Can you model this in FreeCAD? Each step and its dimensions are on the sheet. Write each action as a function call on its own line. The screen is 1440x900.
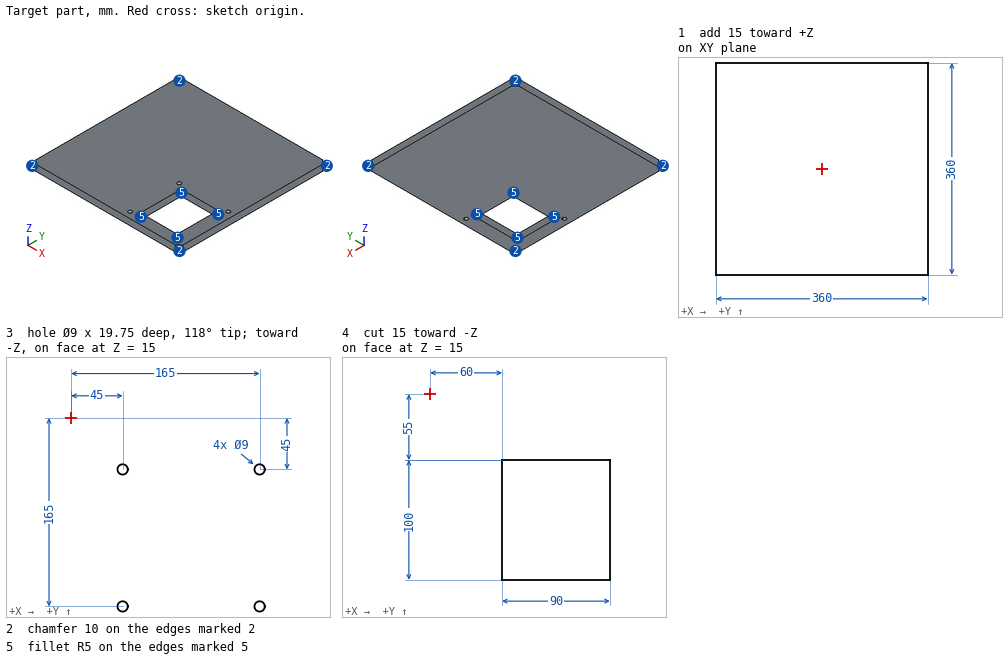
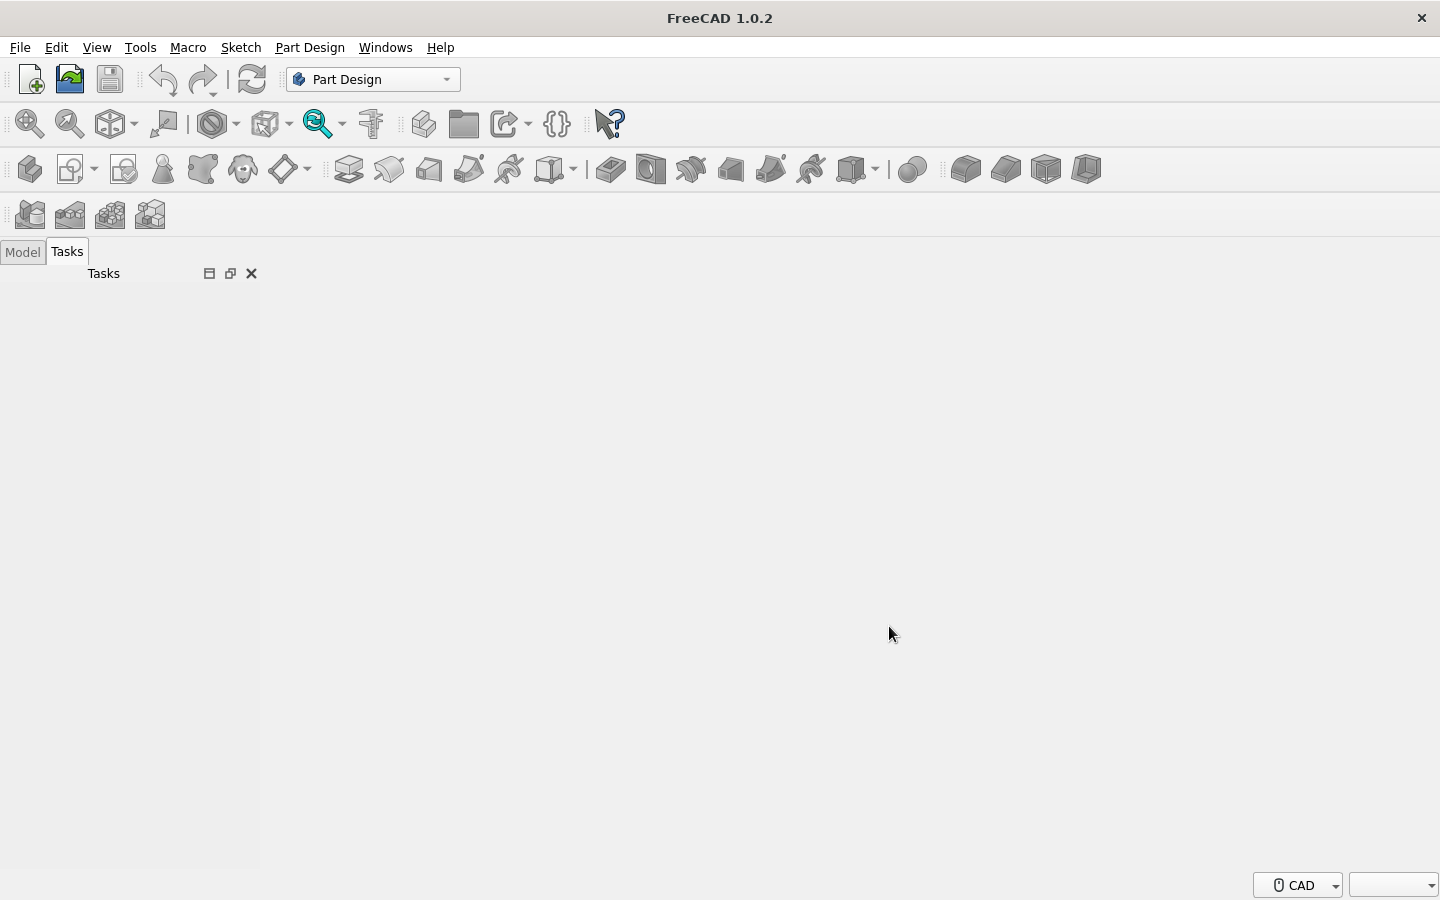
key(ctrl+n)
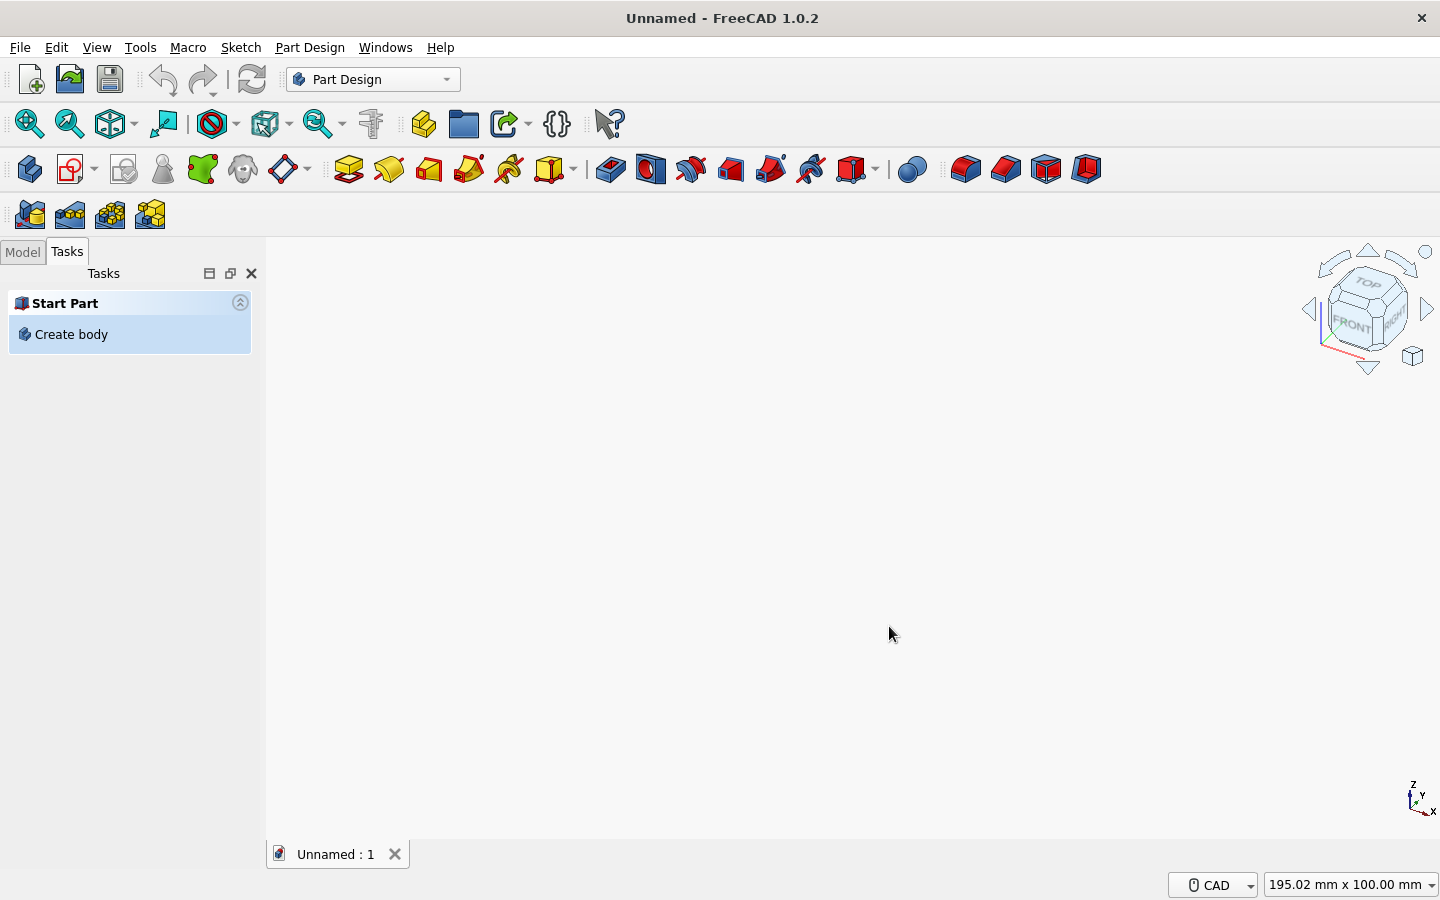
click(70, 170)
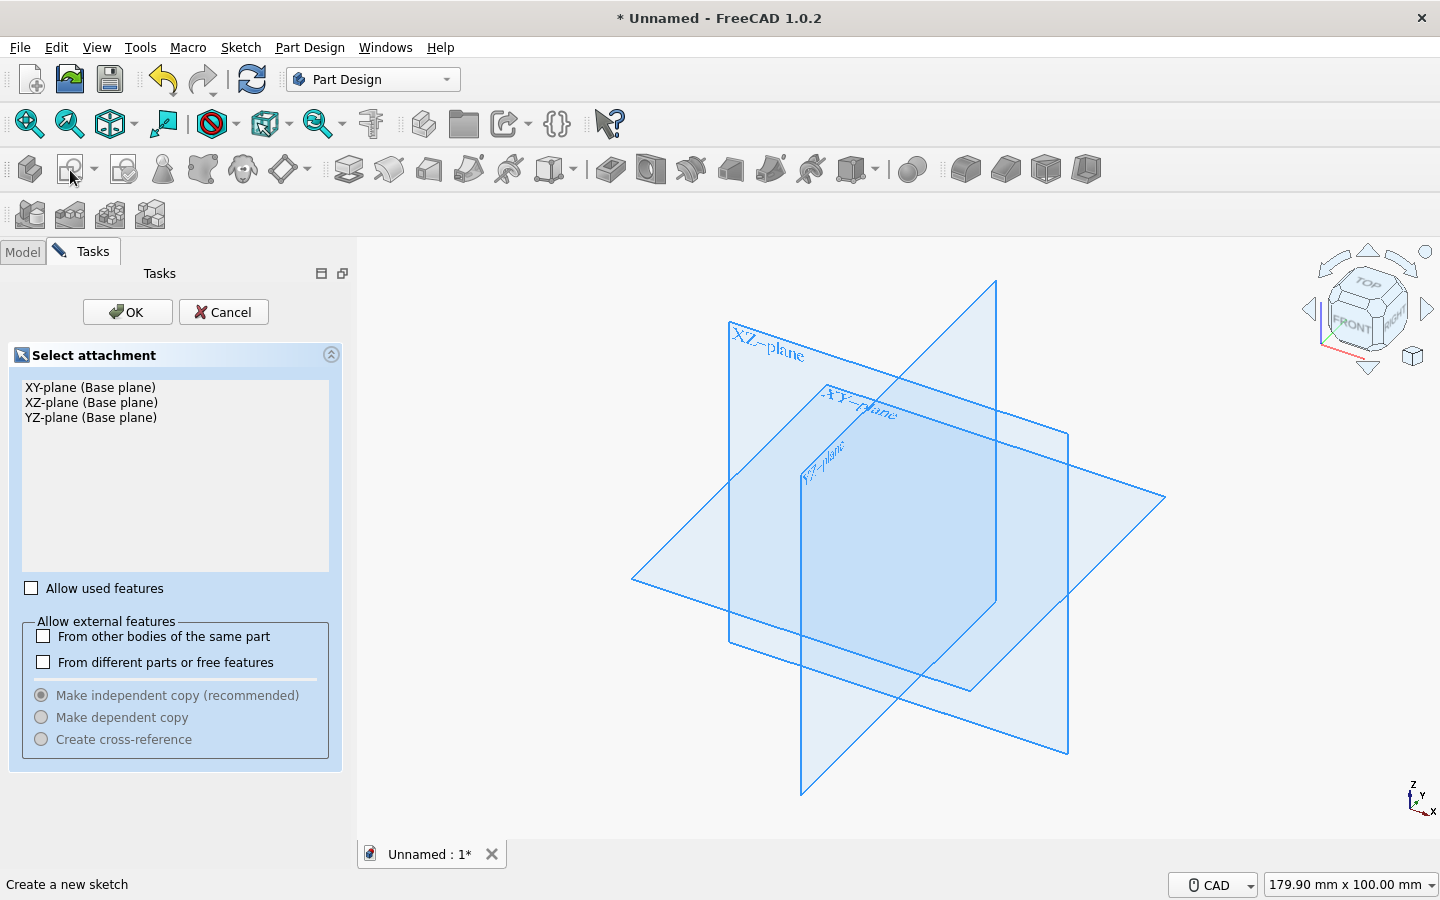
click(82, 388)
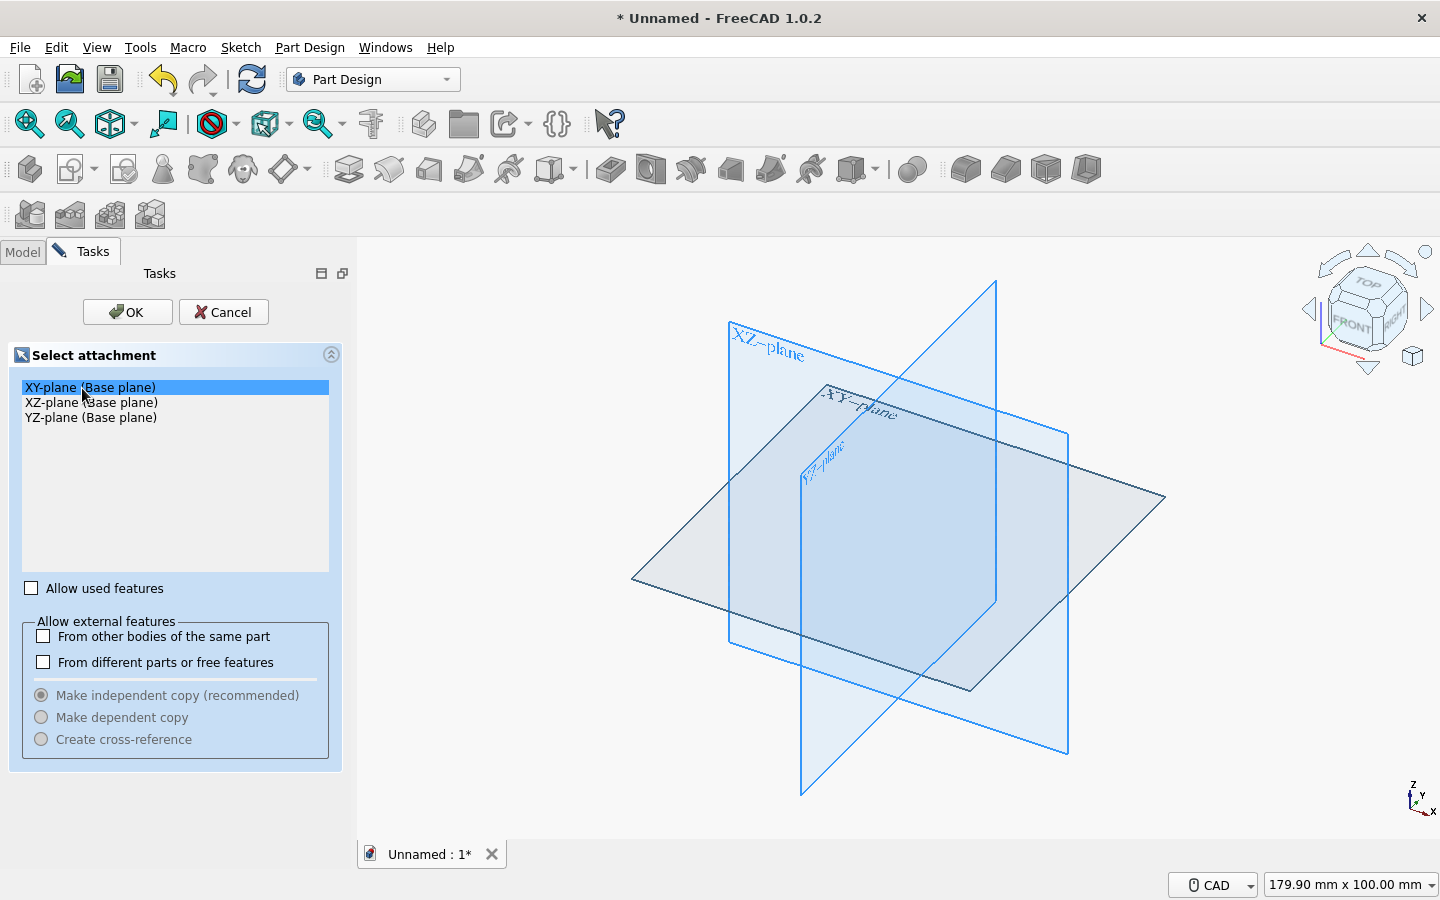
click(128, 312)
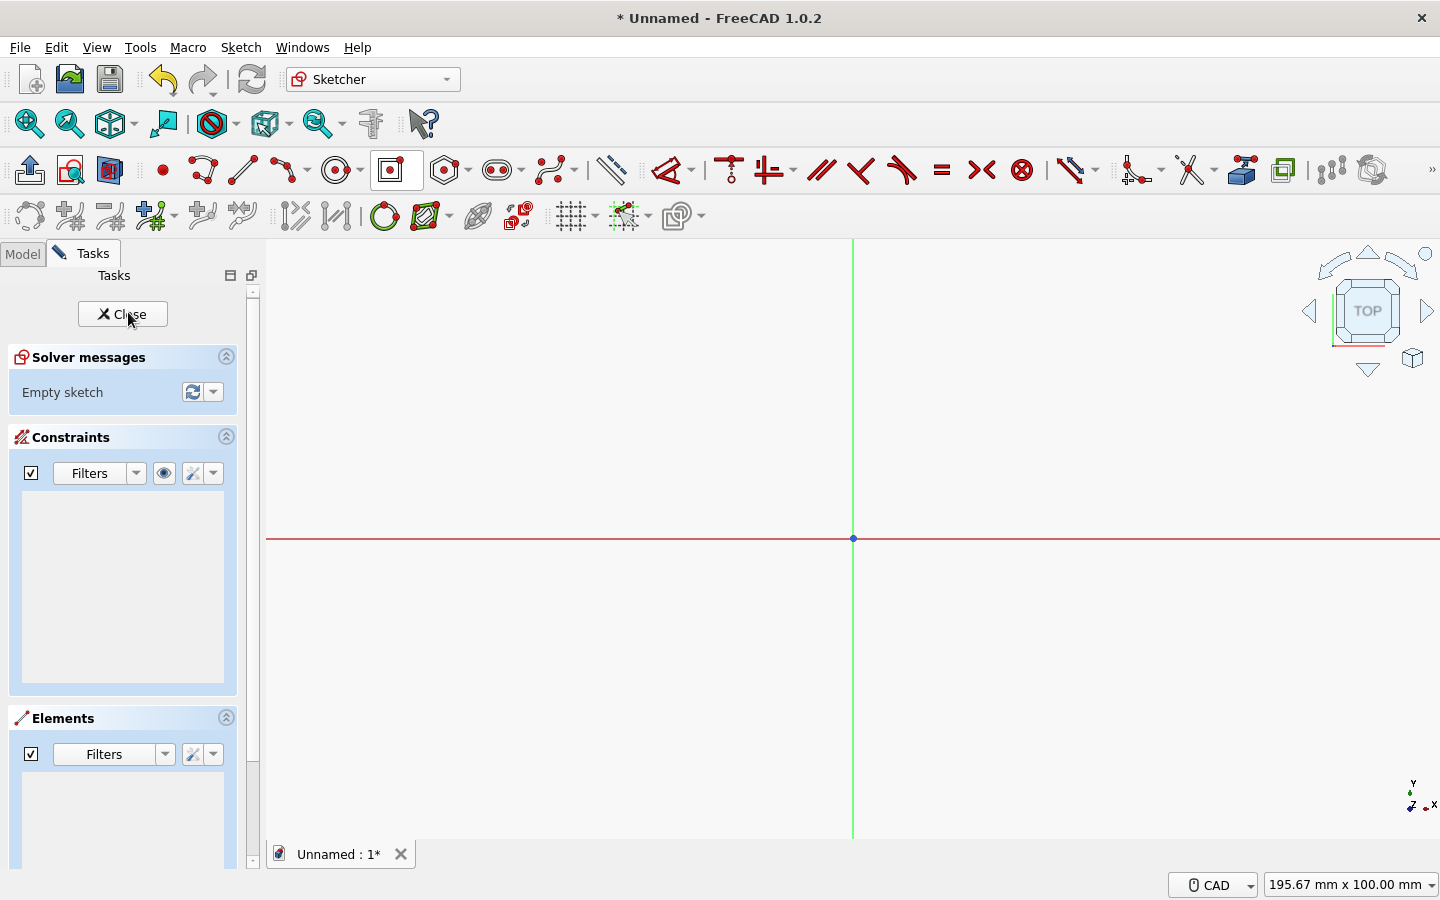
scroll(771, 539, down, 9)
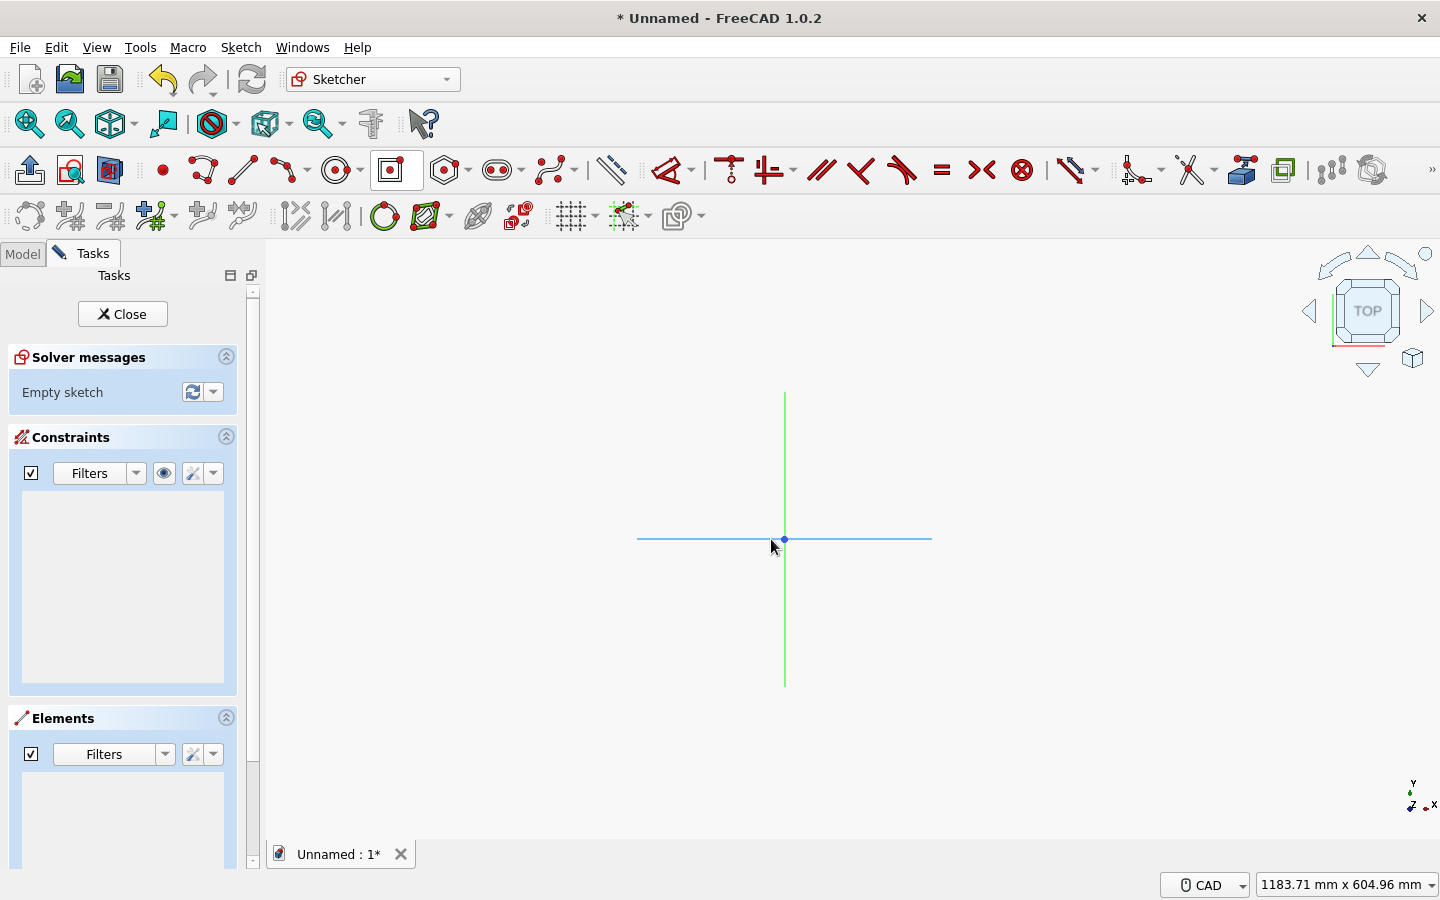
key(g)
key(v)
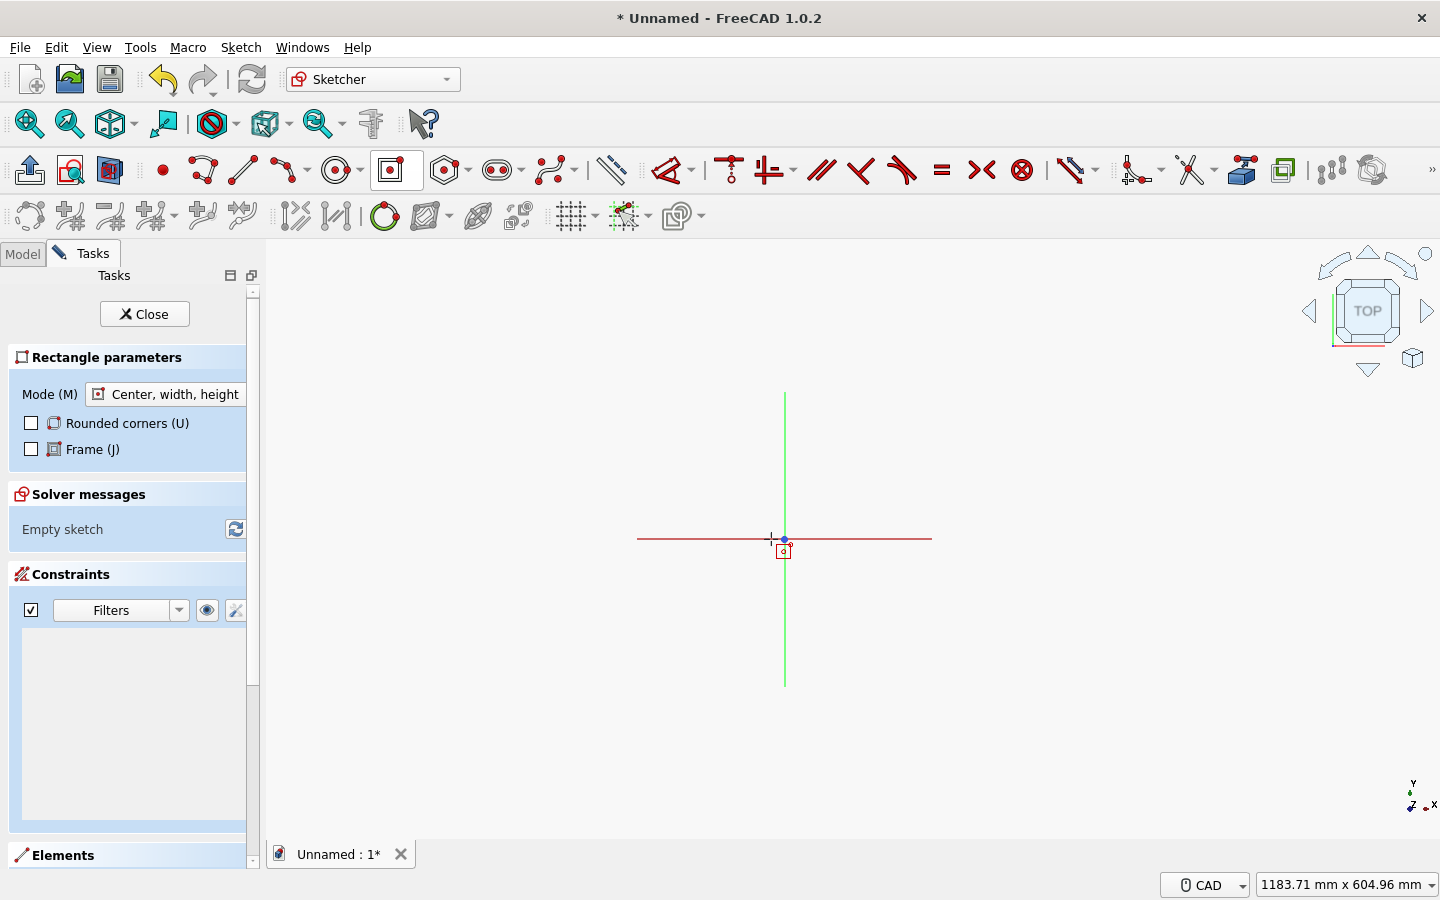
click(785, 539)
click(963, 361)
key(Escape)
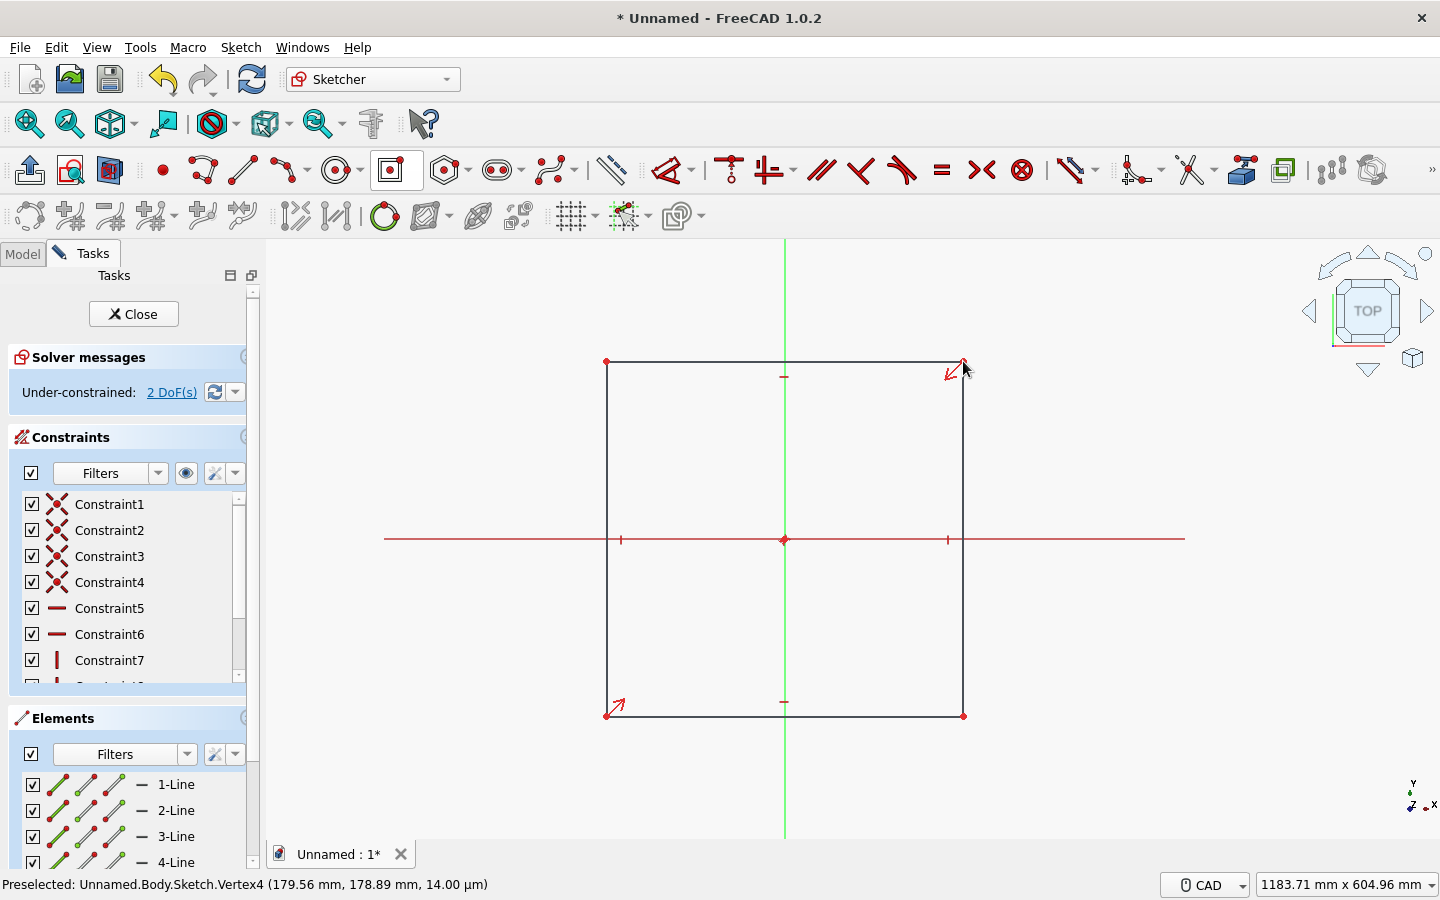
key(d)